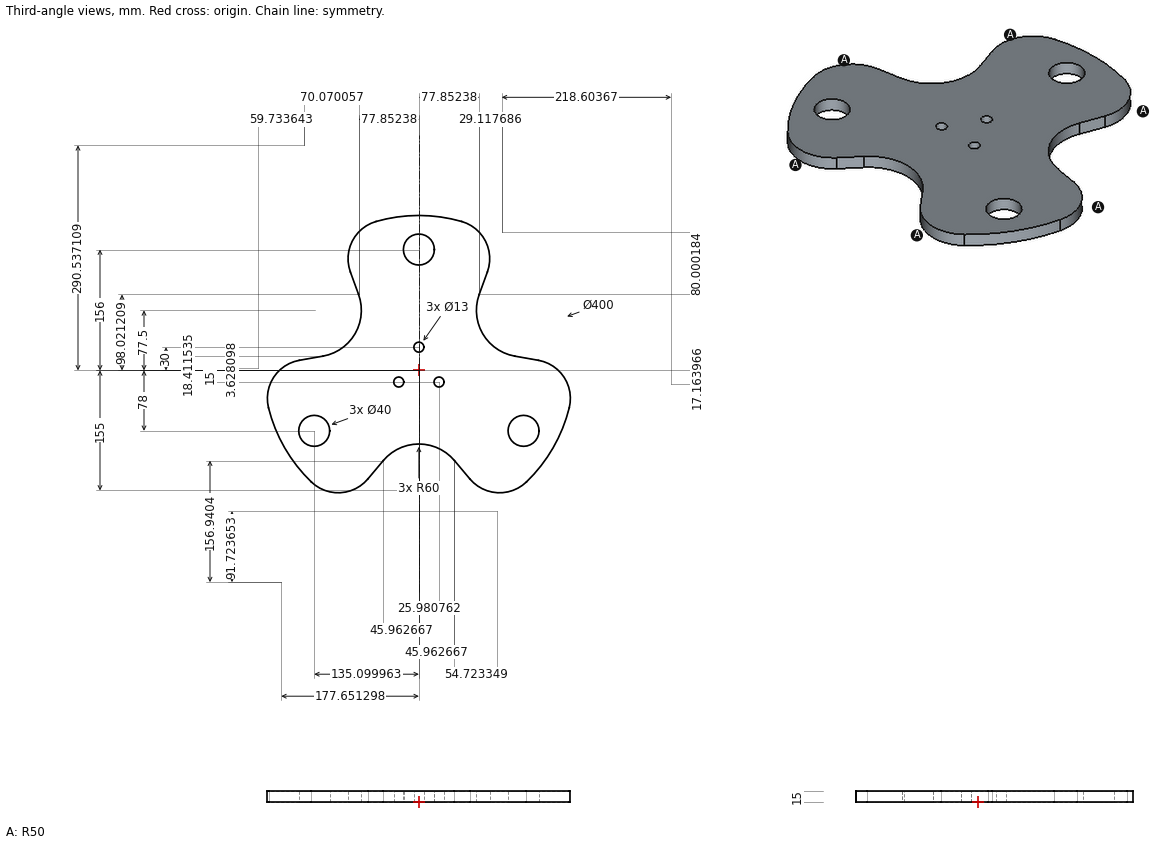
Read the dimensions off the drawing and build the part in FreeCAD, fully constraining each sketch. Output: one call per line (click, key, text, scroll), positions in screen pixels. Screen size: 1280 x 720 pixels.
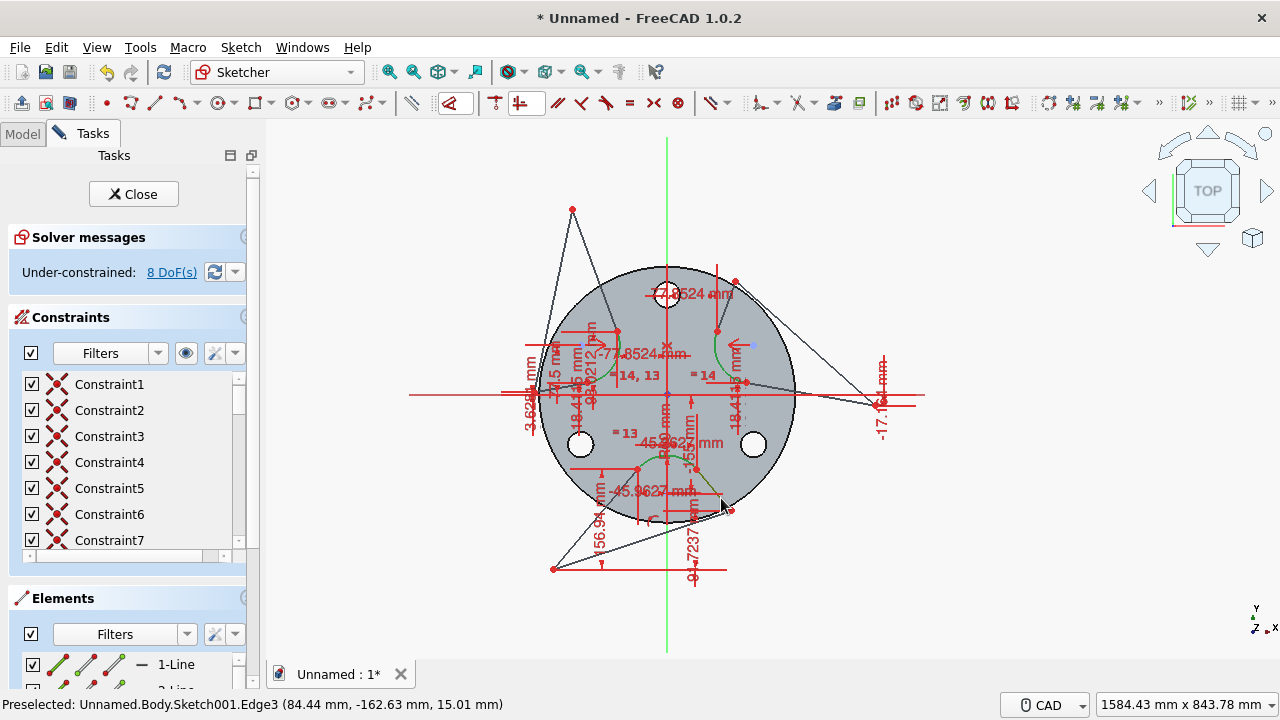
key(l)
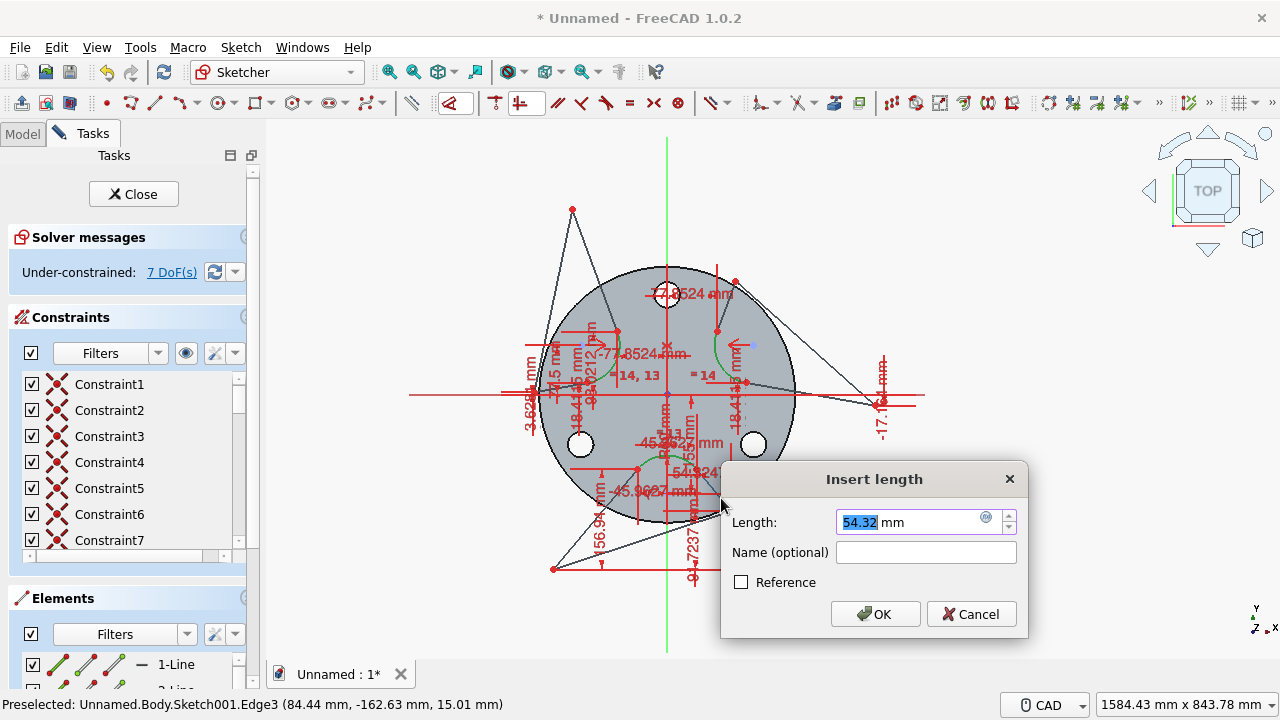
text(54.723349)
key(Return)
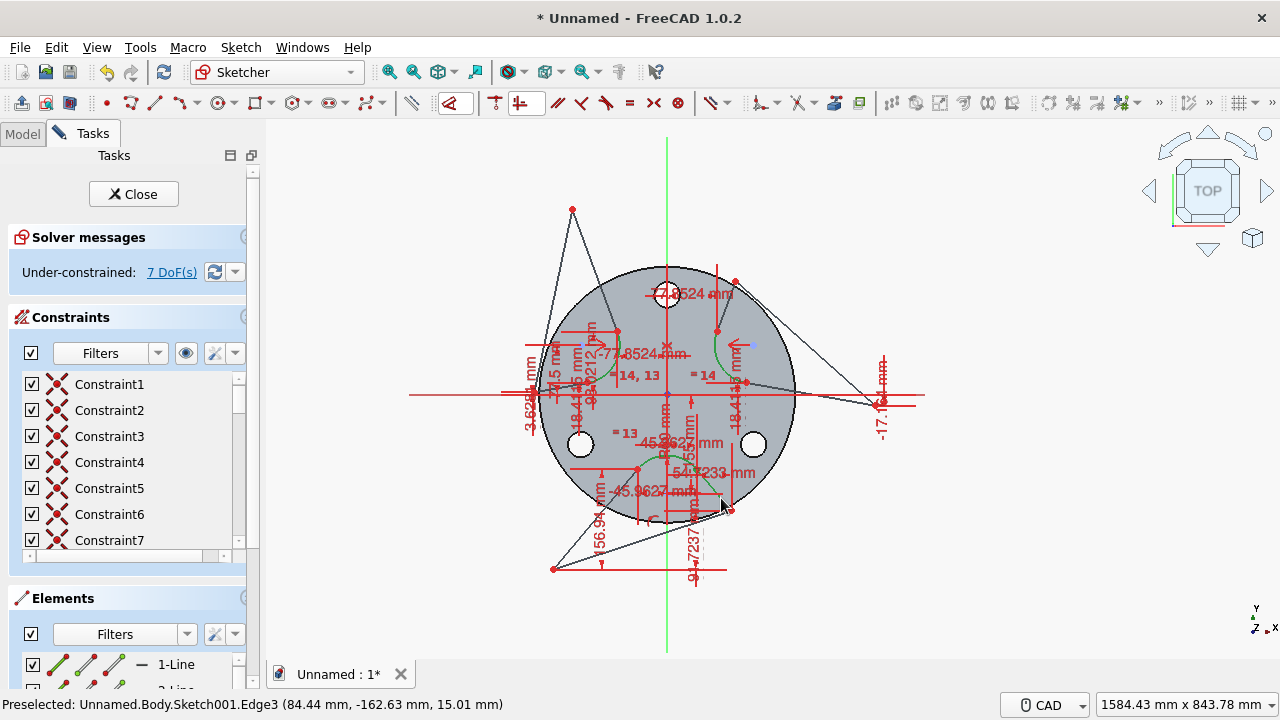
click(604, 295)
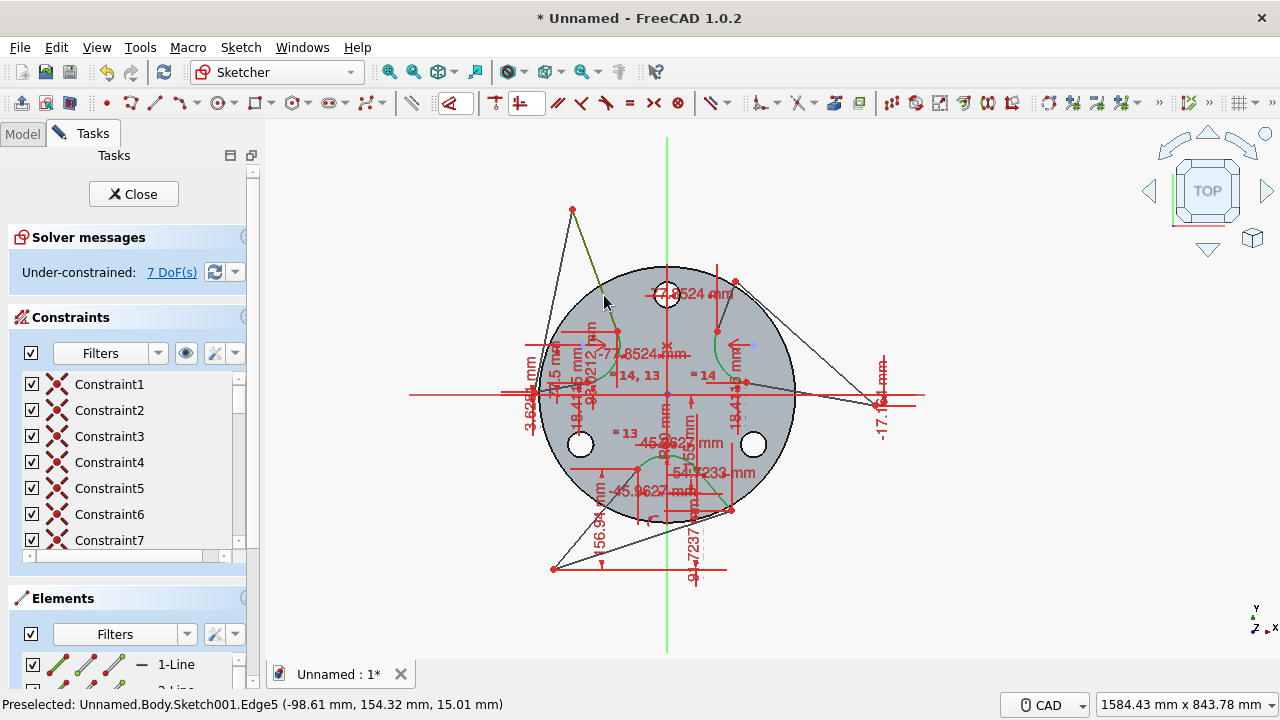
click(468, 104)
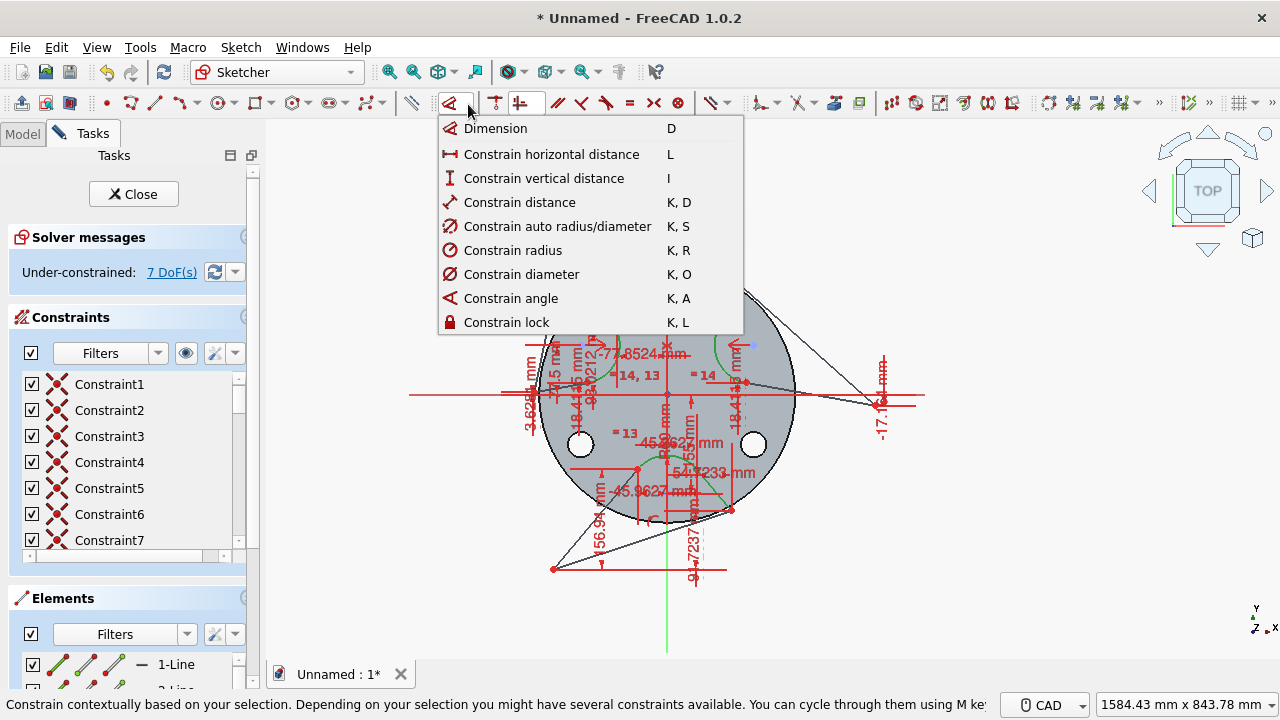
click(591, 154)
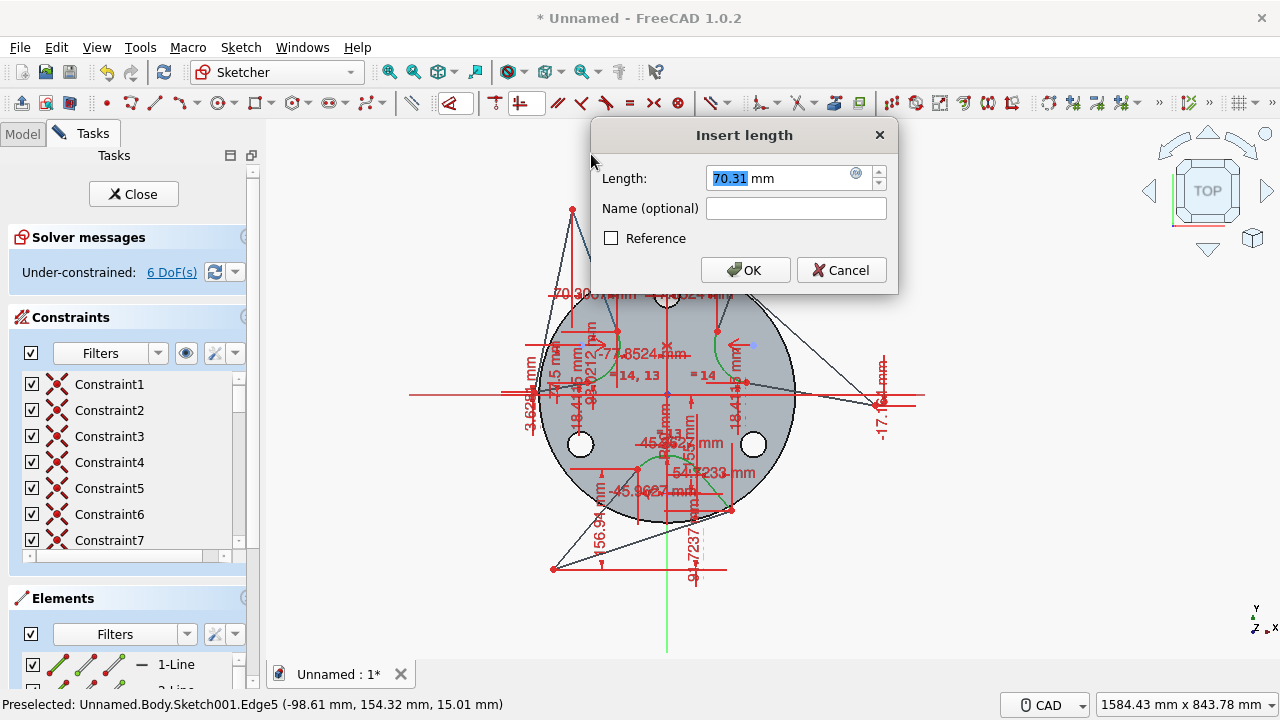
text(70.070057)
key(Return)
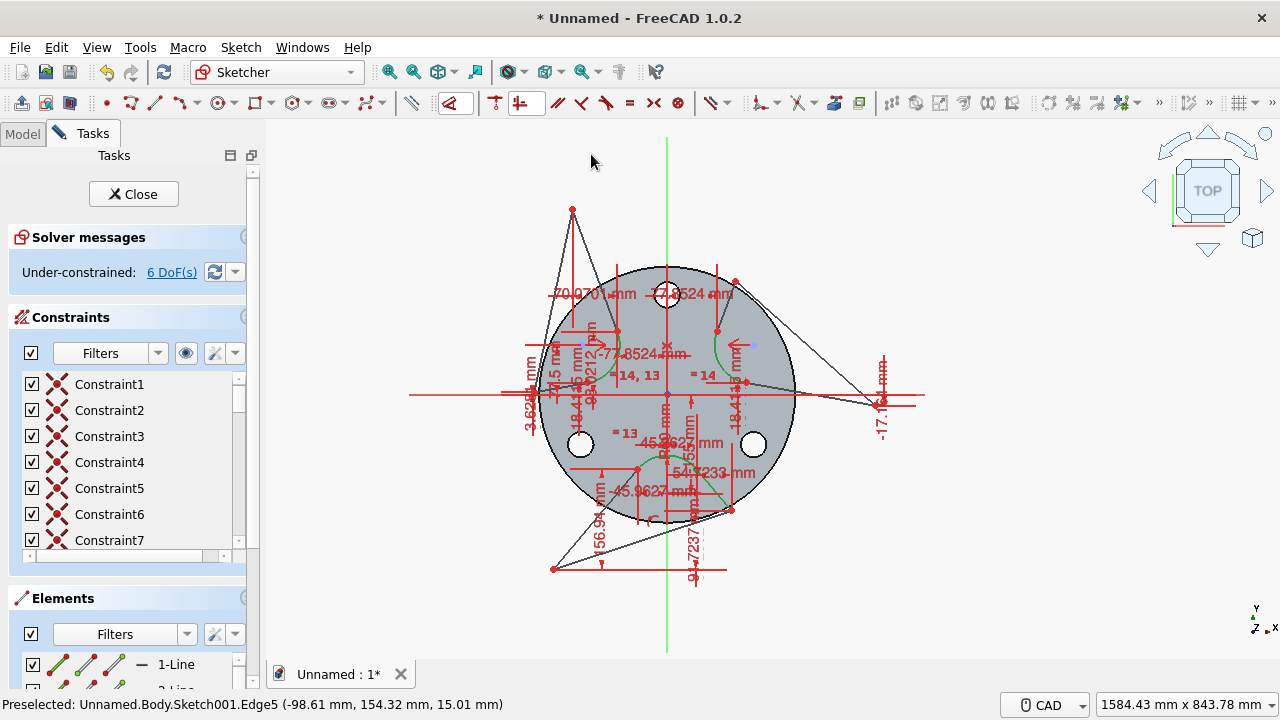
click(561, 265)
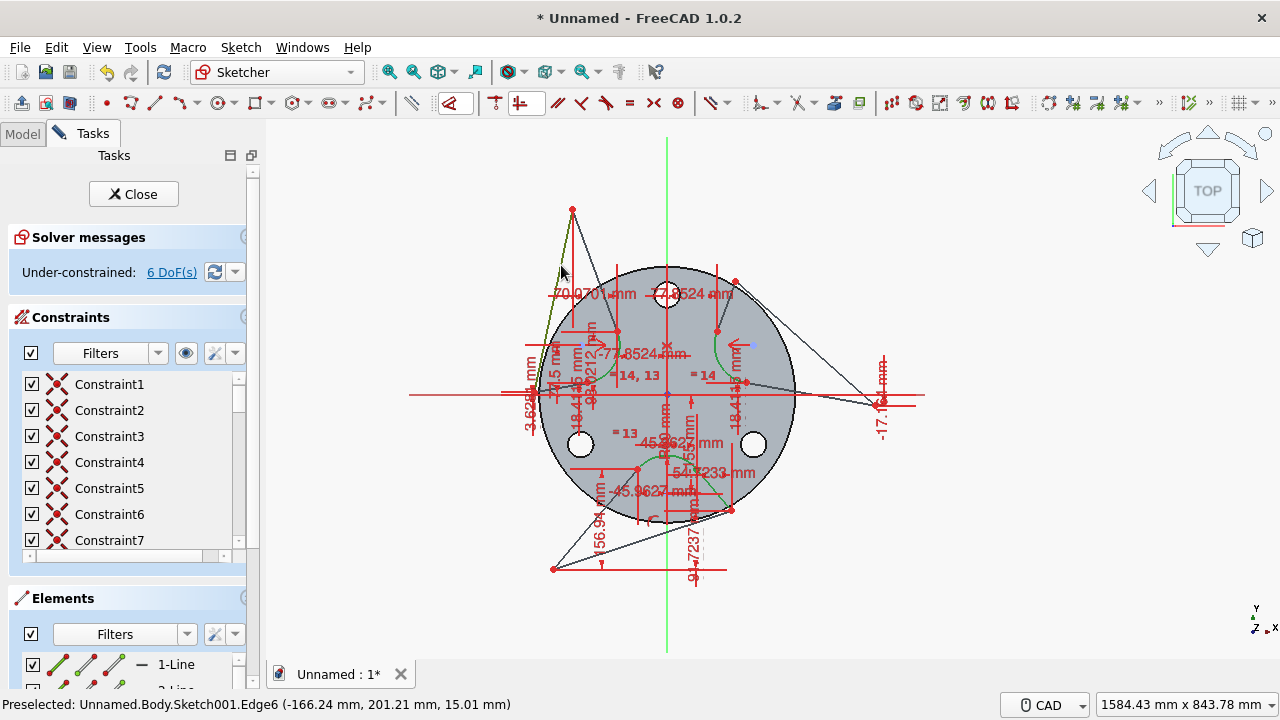
click(468, 104)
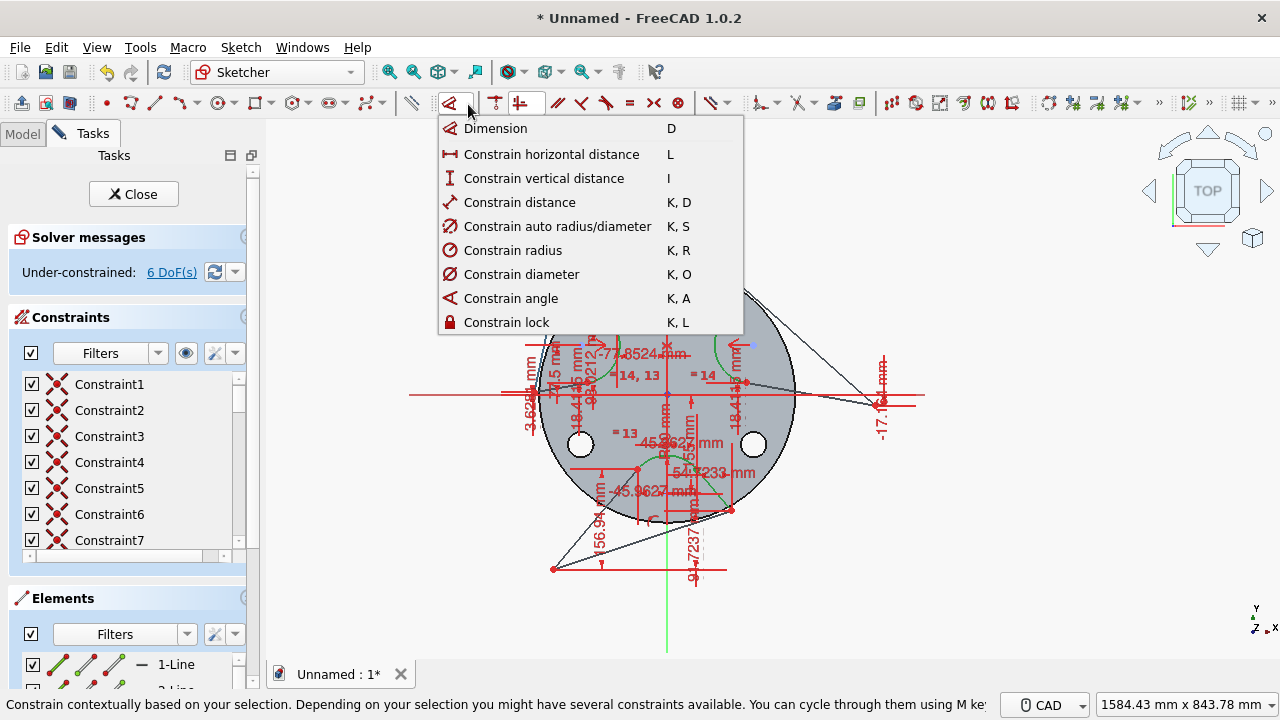
click(591, 154)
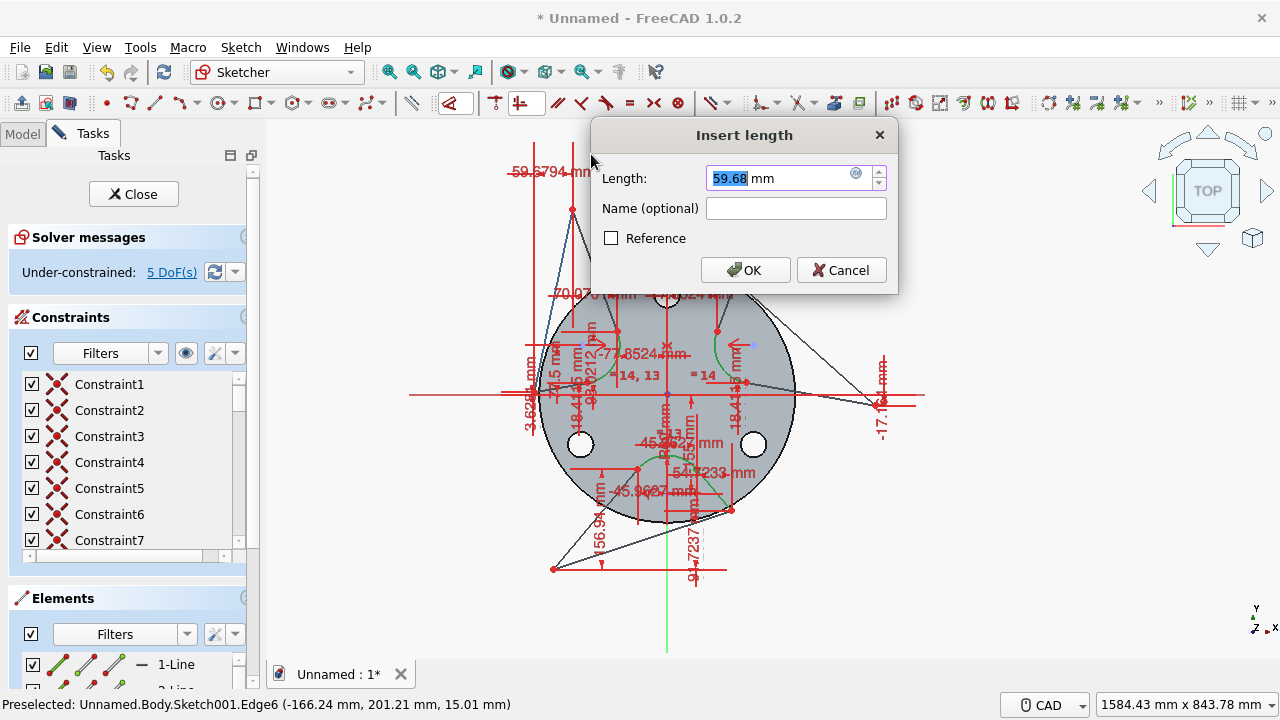
text(59.733643)
key(Return)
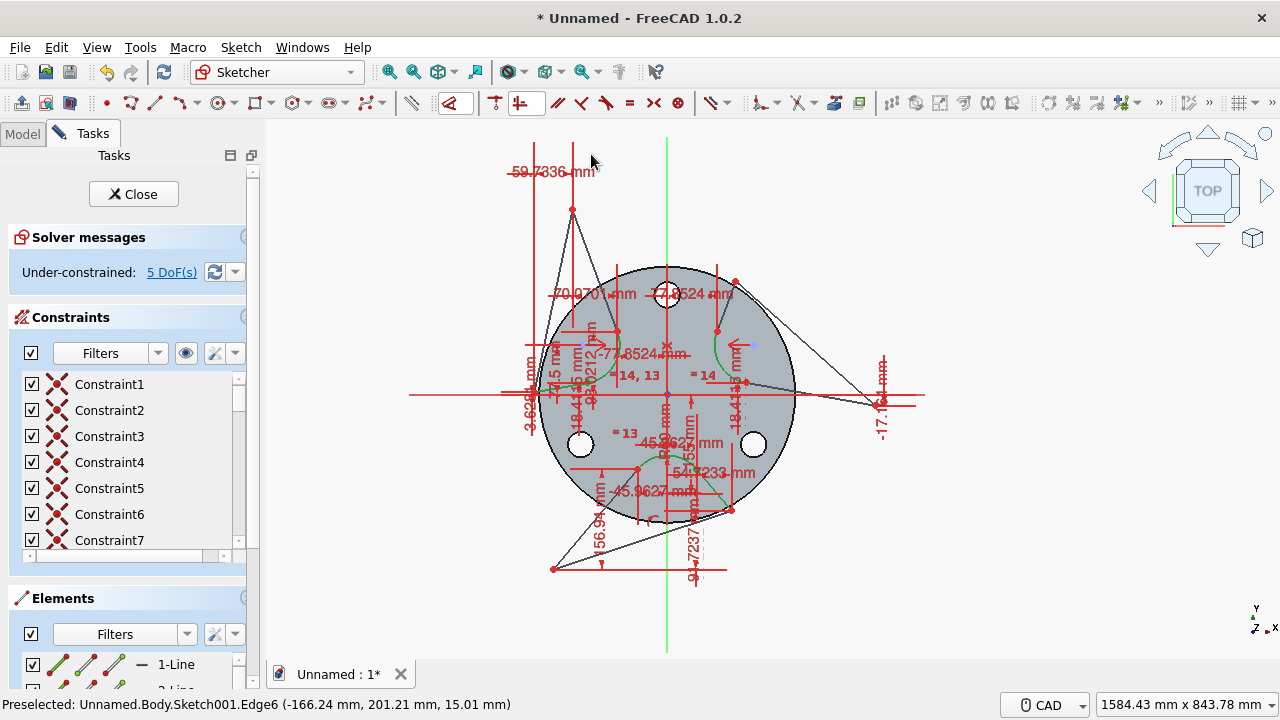
click(834, 368)